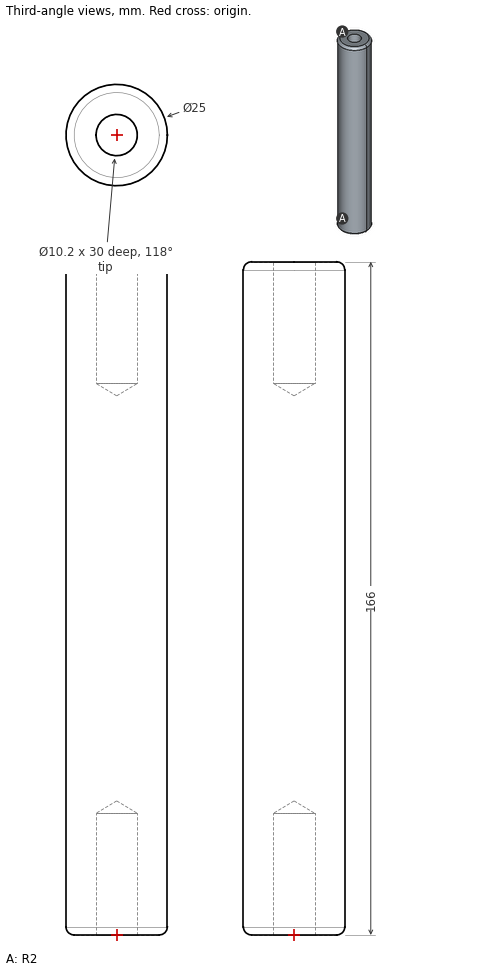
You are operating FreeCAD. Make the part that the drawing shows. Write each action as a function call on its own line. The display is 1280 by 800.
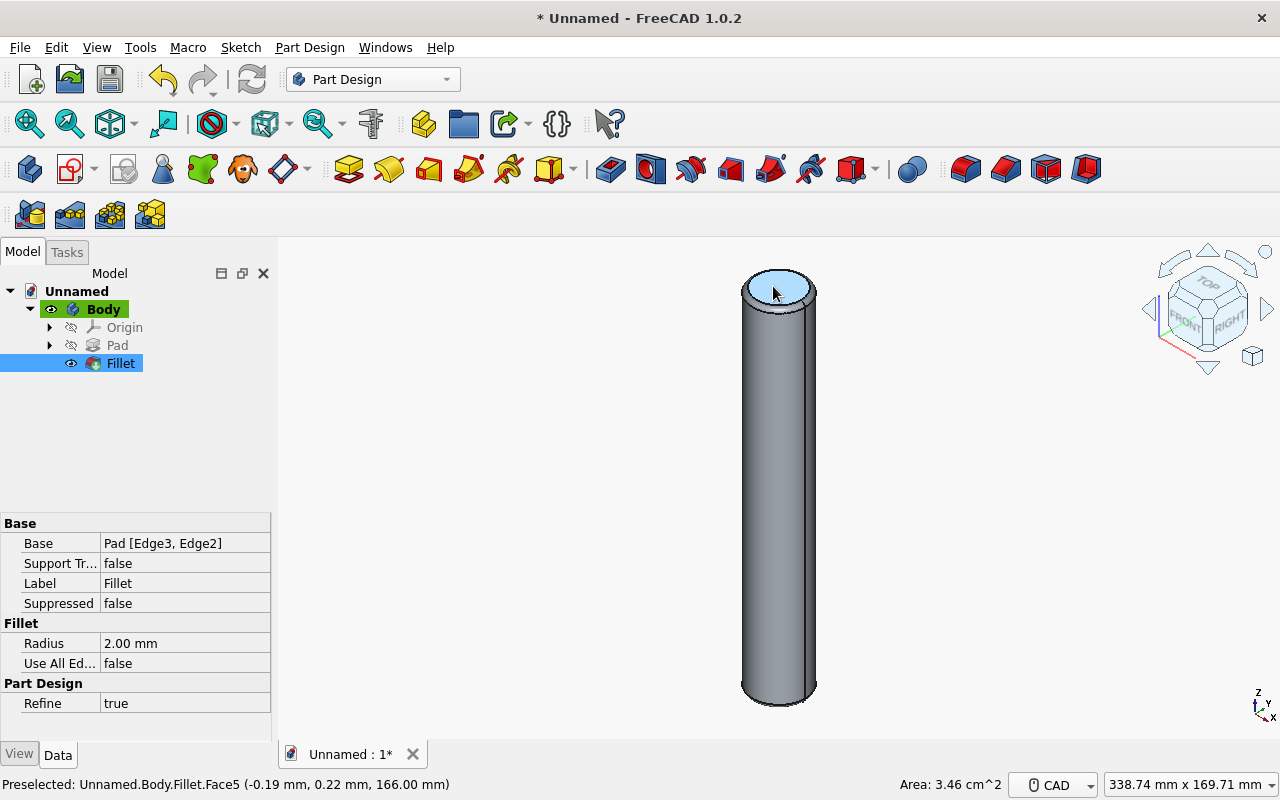
click(70, 170)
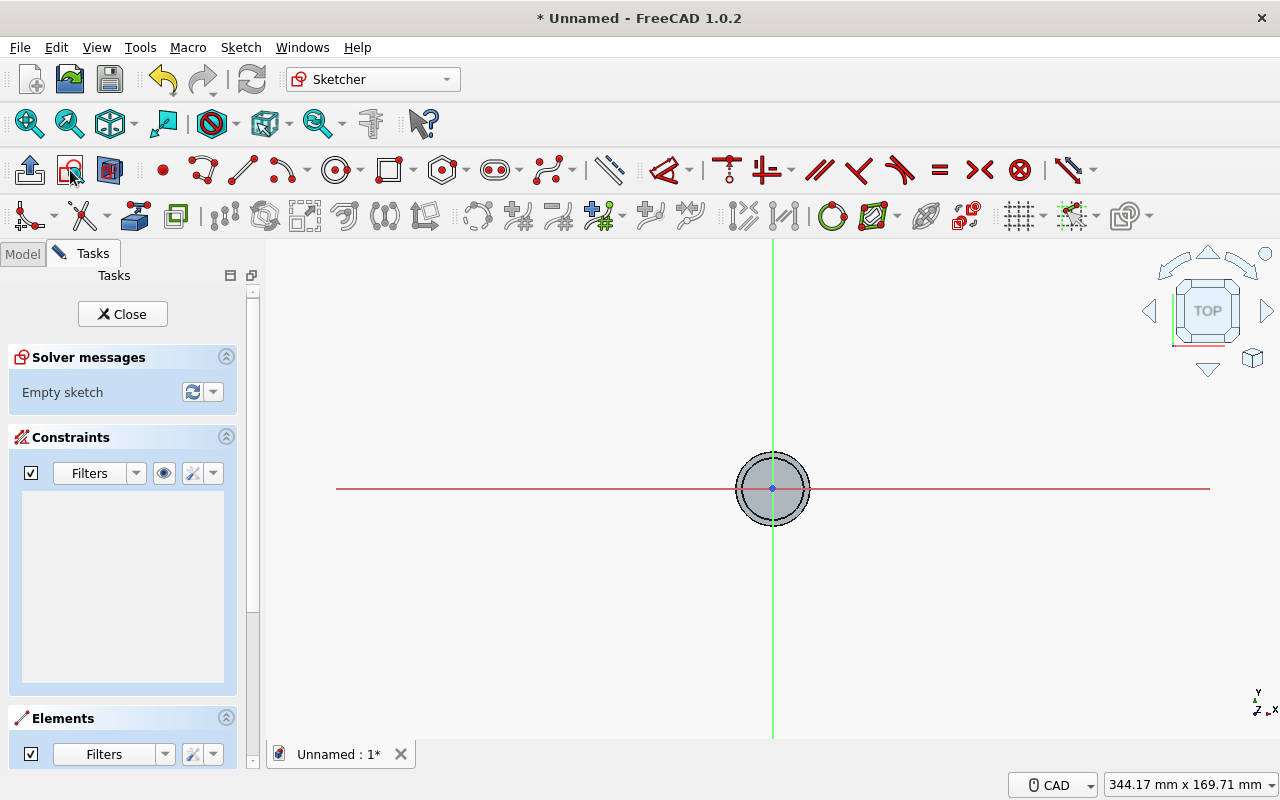
scroll(780, 489, up, 12)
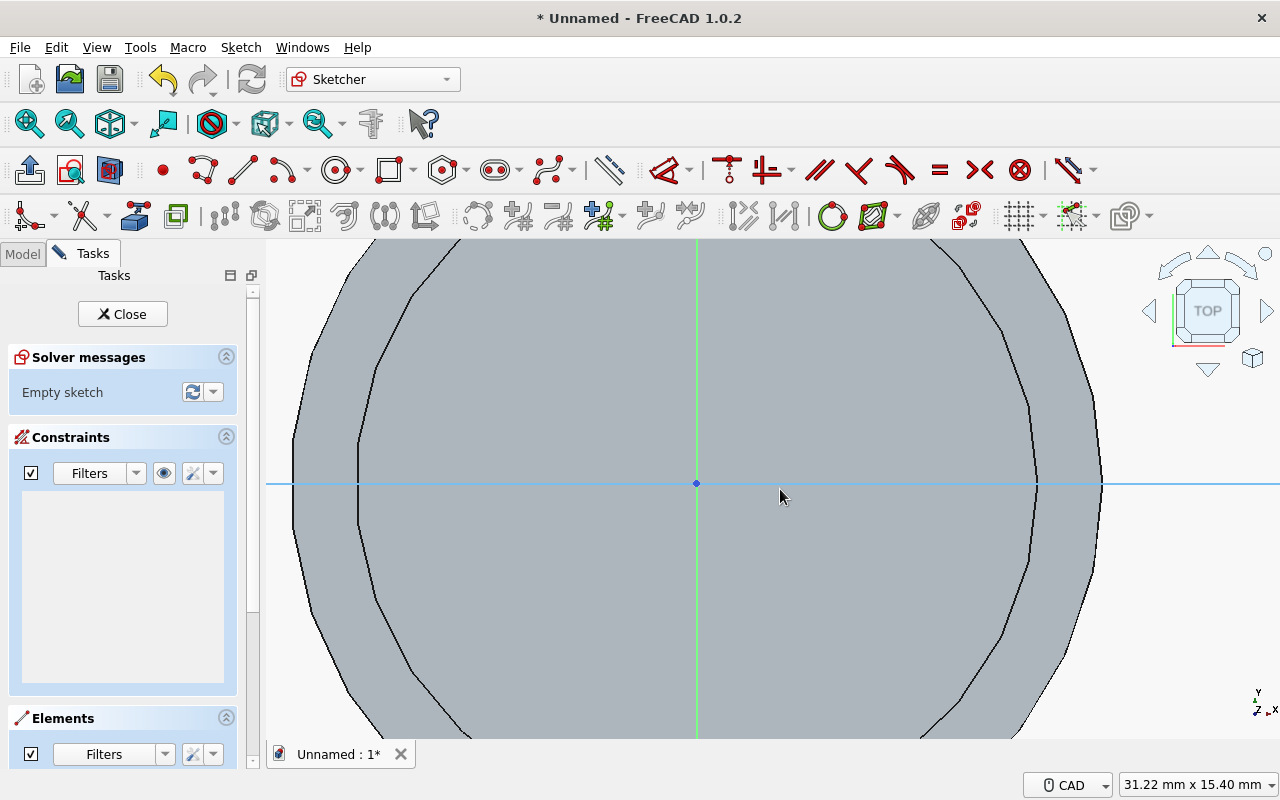
click(336, 170)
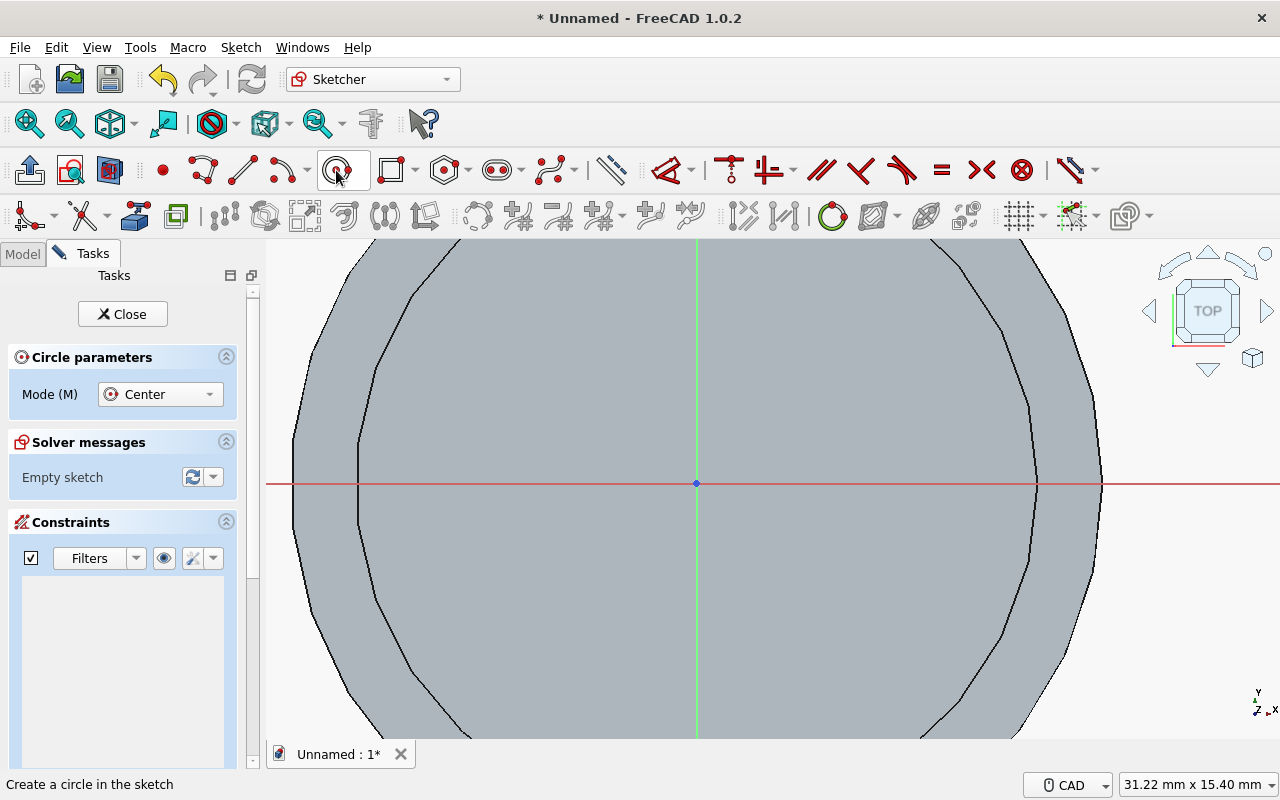
click(697, 484)
click(814, 367)
key(Escape)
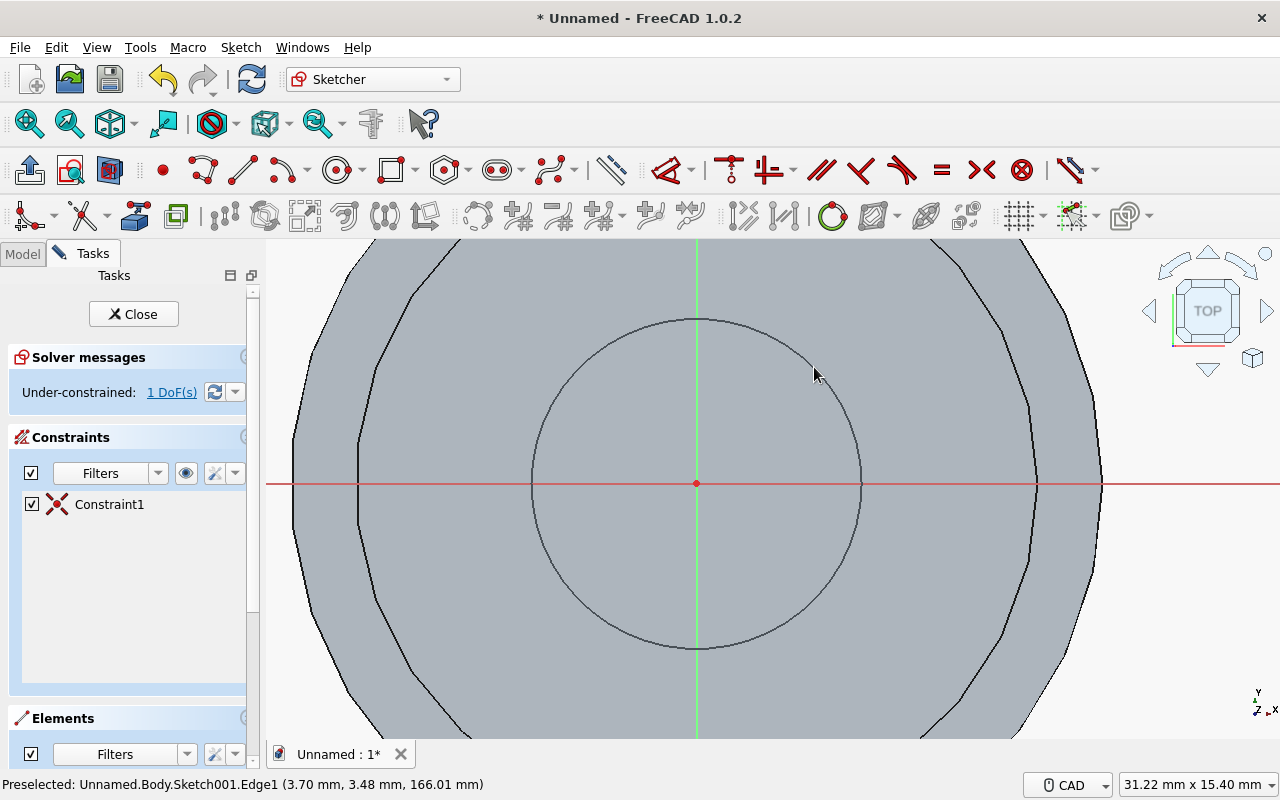
click(666, 170)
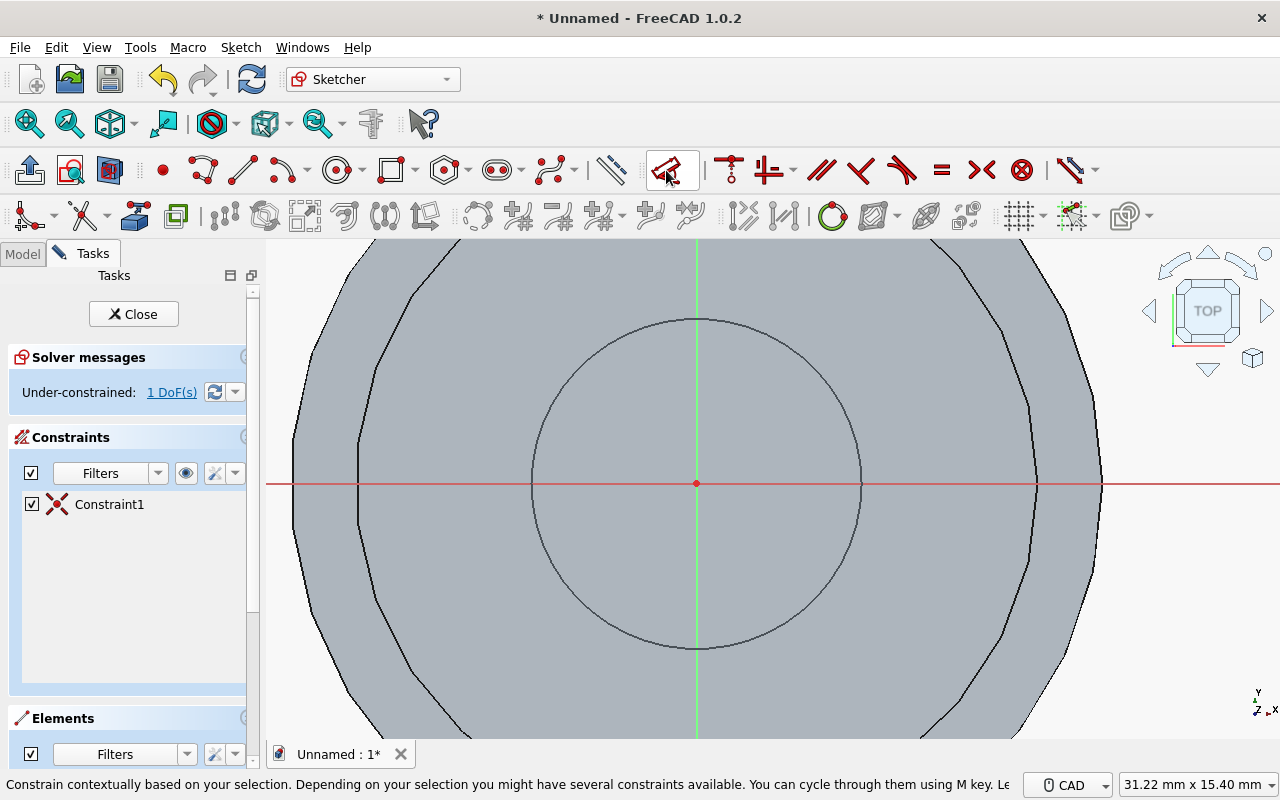
click(813, 367)
click(836, 344)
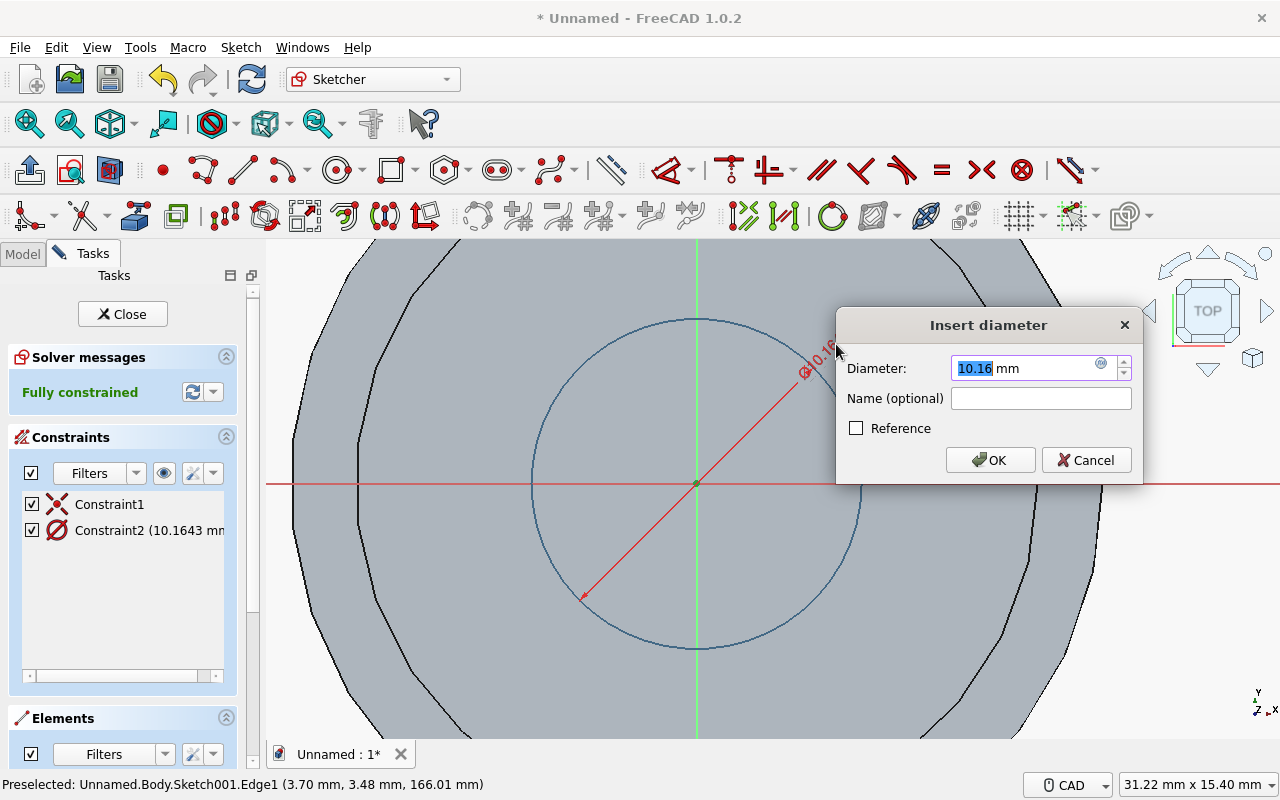
text(10.2)
key(Return)
key(Escape)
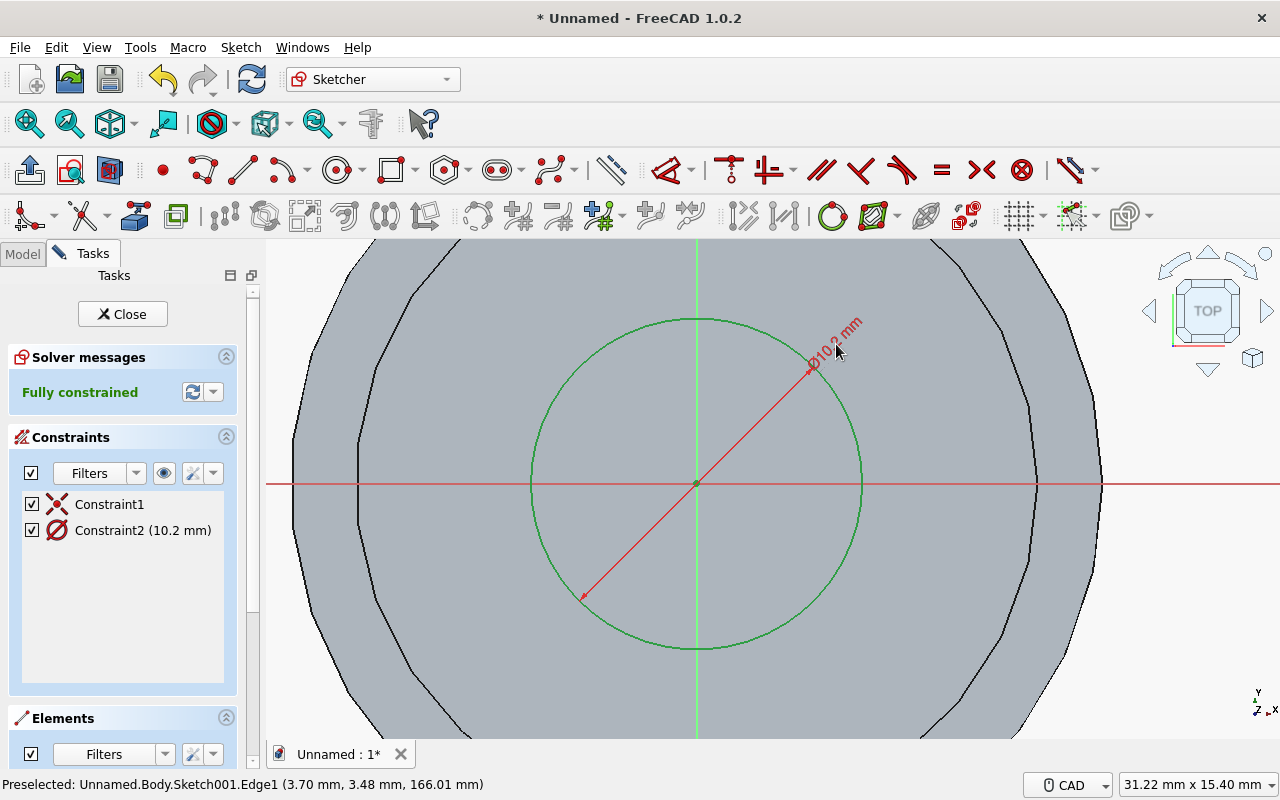
click(123, 314)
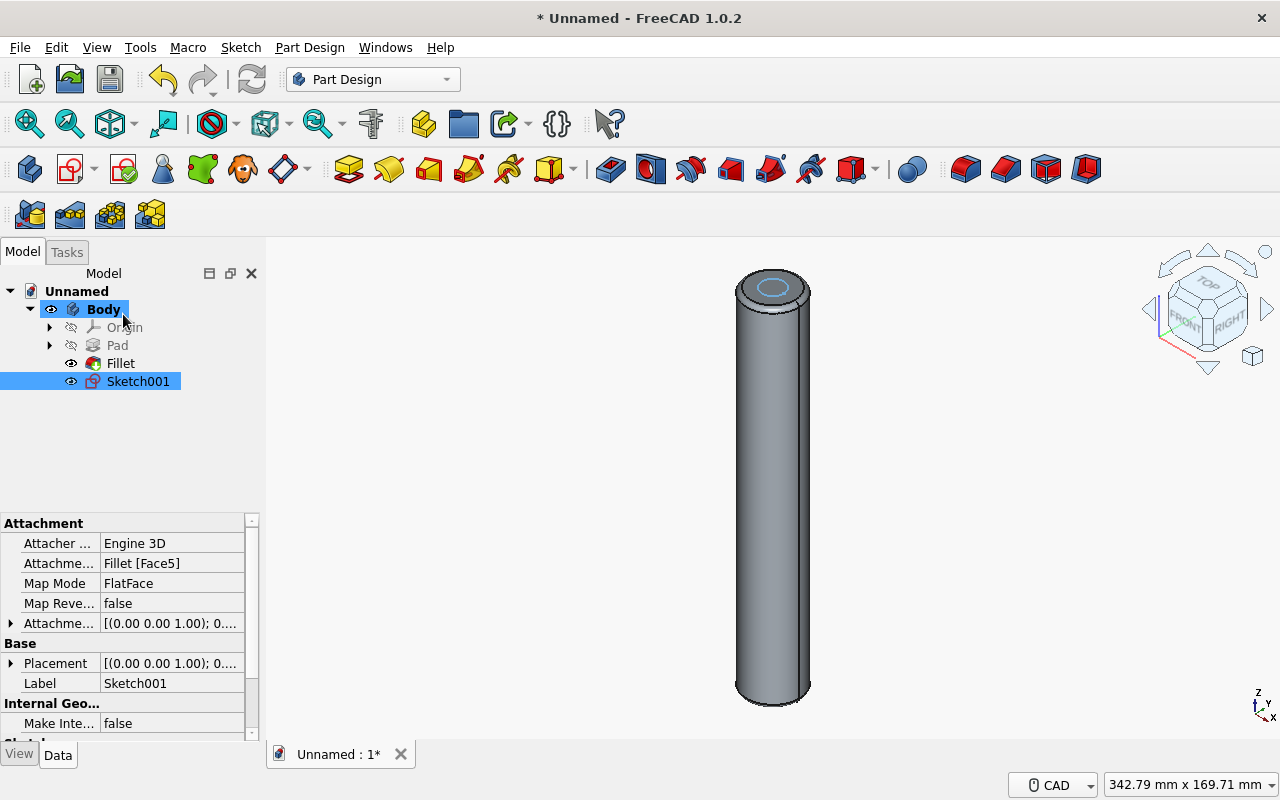
click(652, 170)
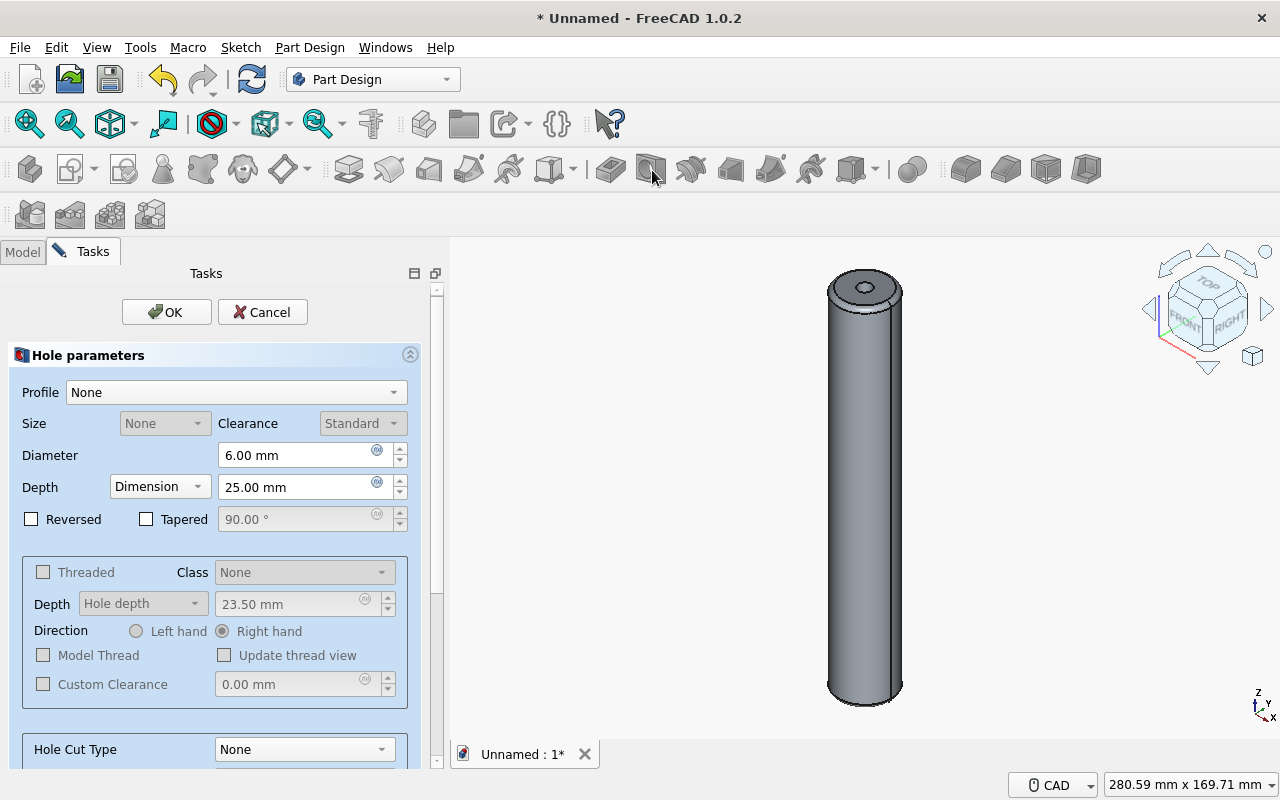
triple_click(305, 455)